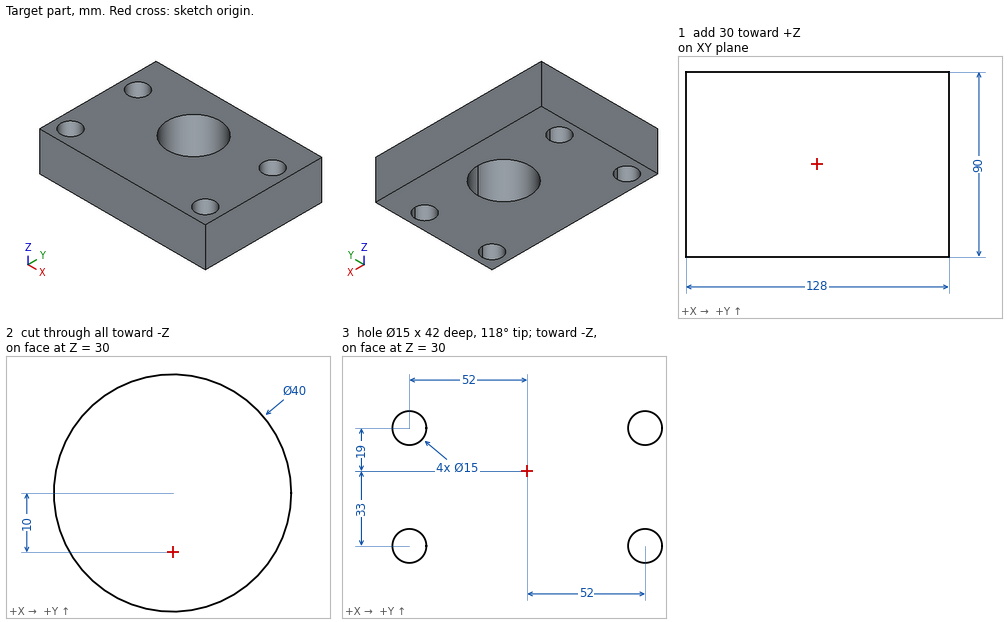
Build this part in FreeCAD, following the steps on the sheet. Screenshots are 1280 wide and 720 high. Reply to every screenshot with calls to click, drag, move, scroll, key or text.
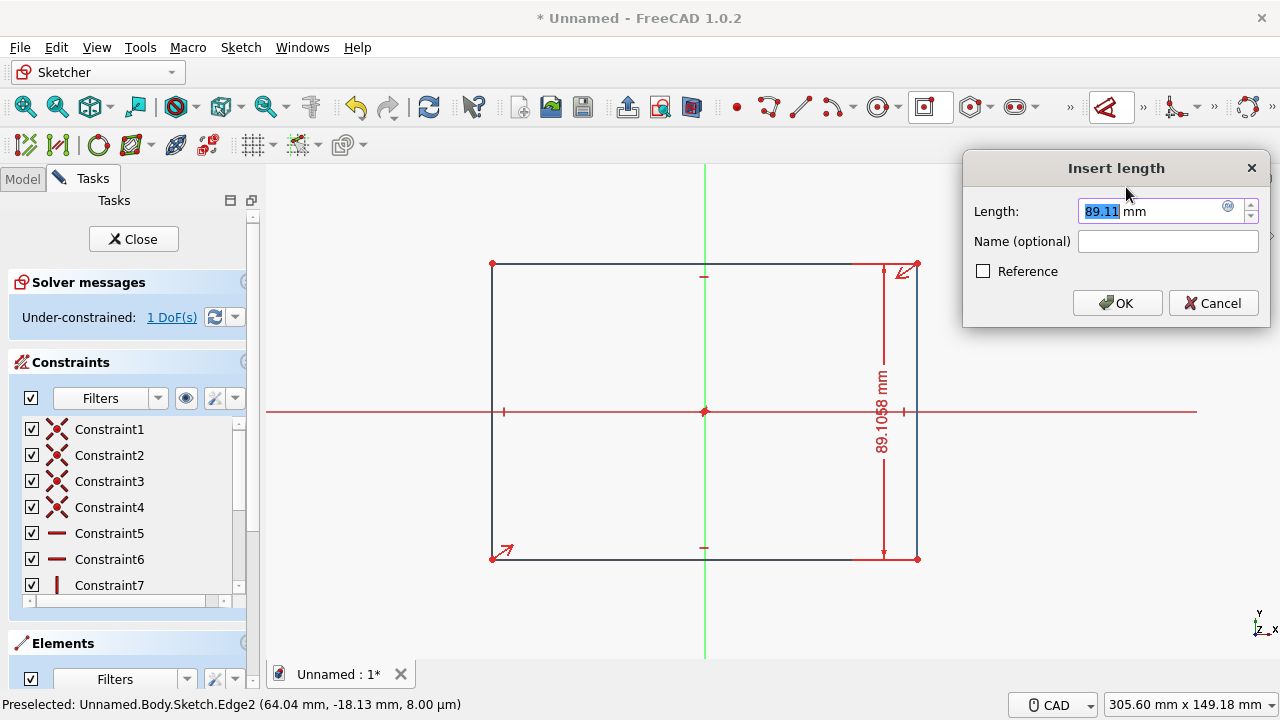
text(90)
key(Return)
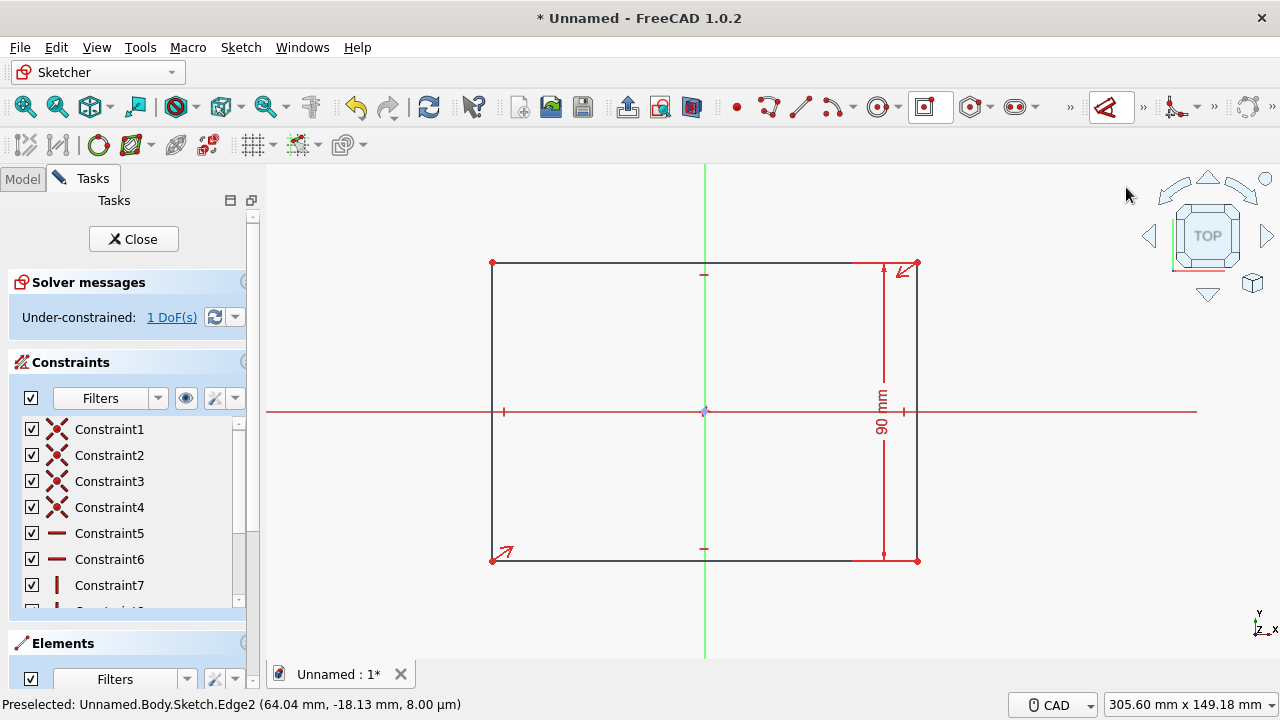
click(620, 561)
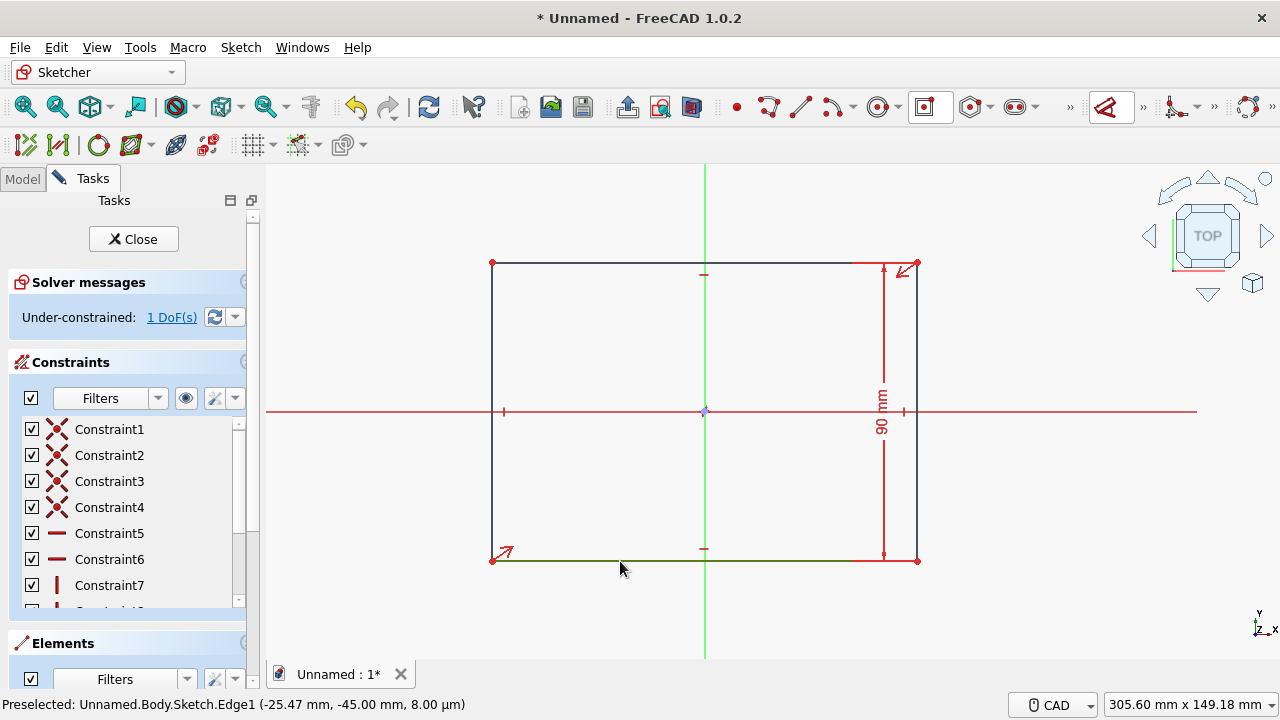
click(1128, 108)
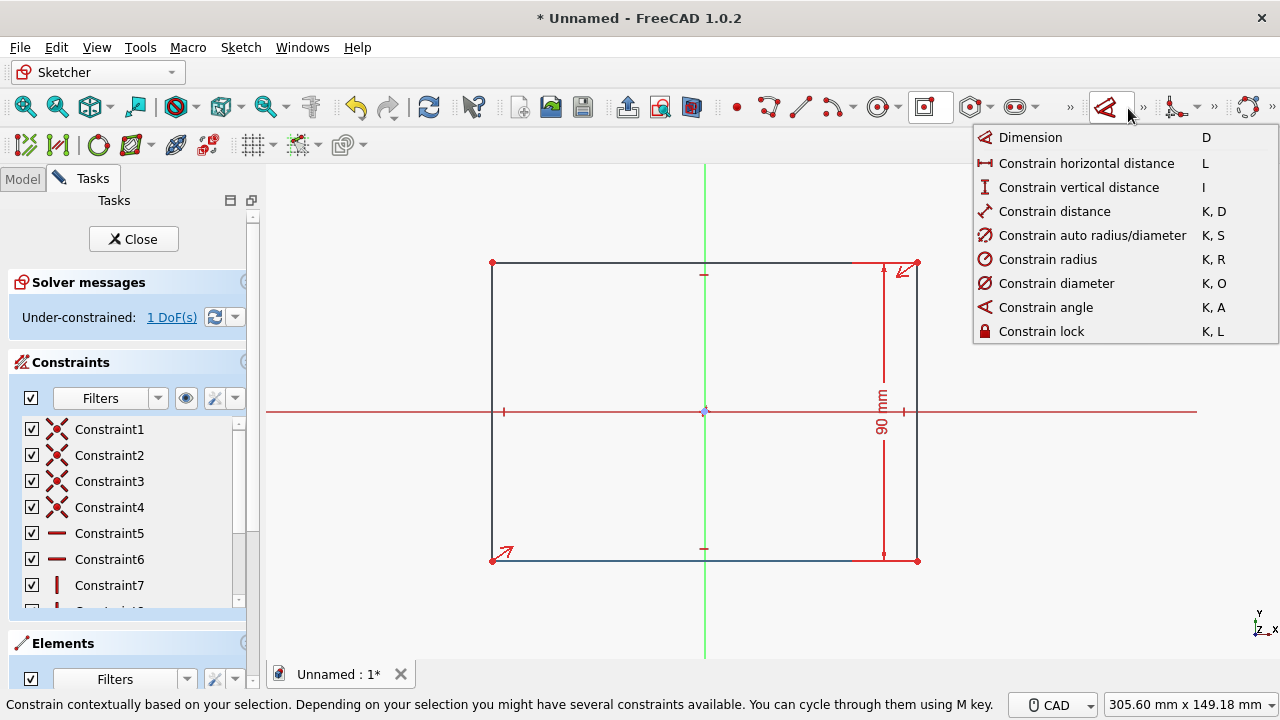
click(1126, 163)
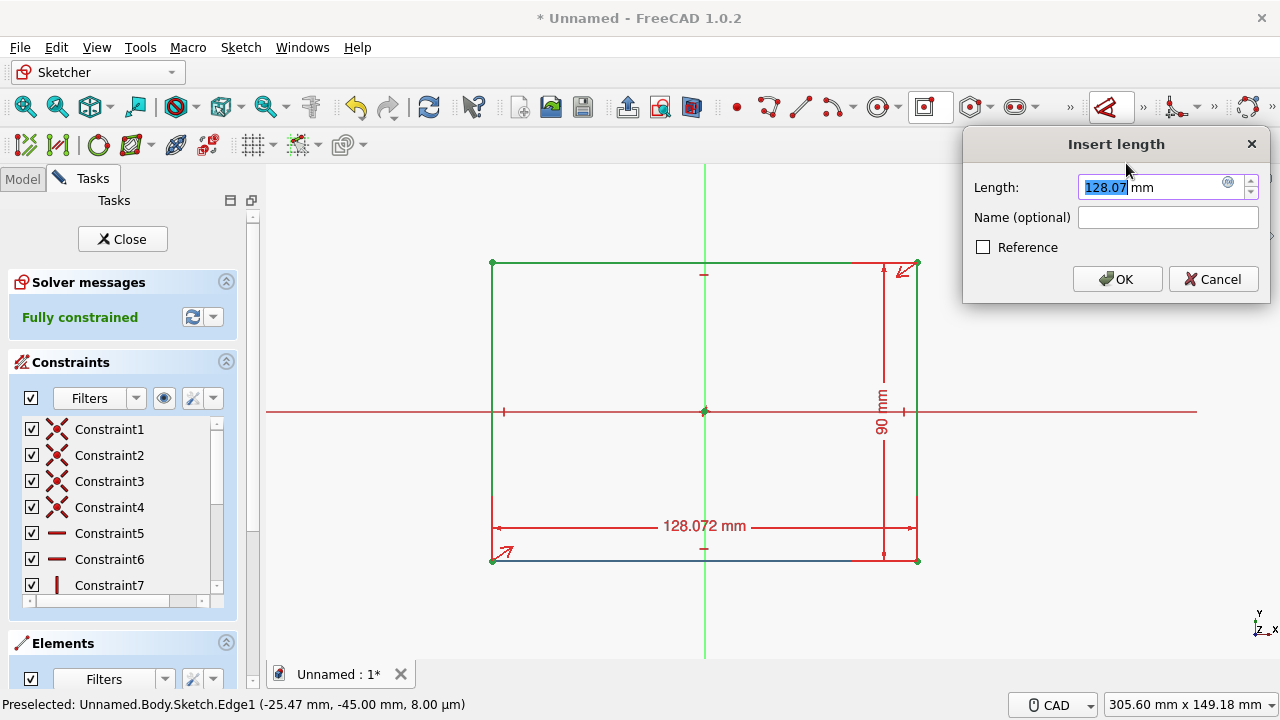
text(128)
key(Return)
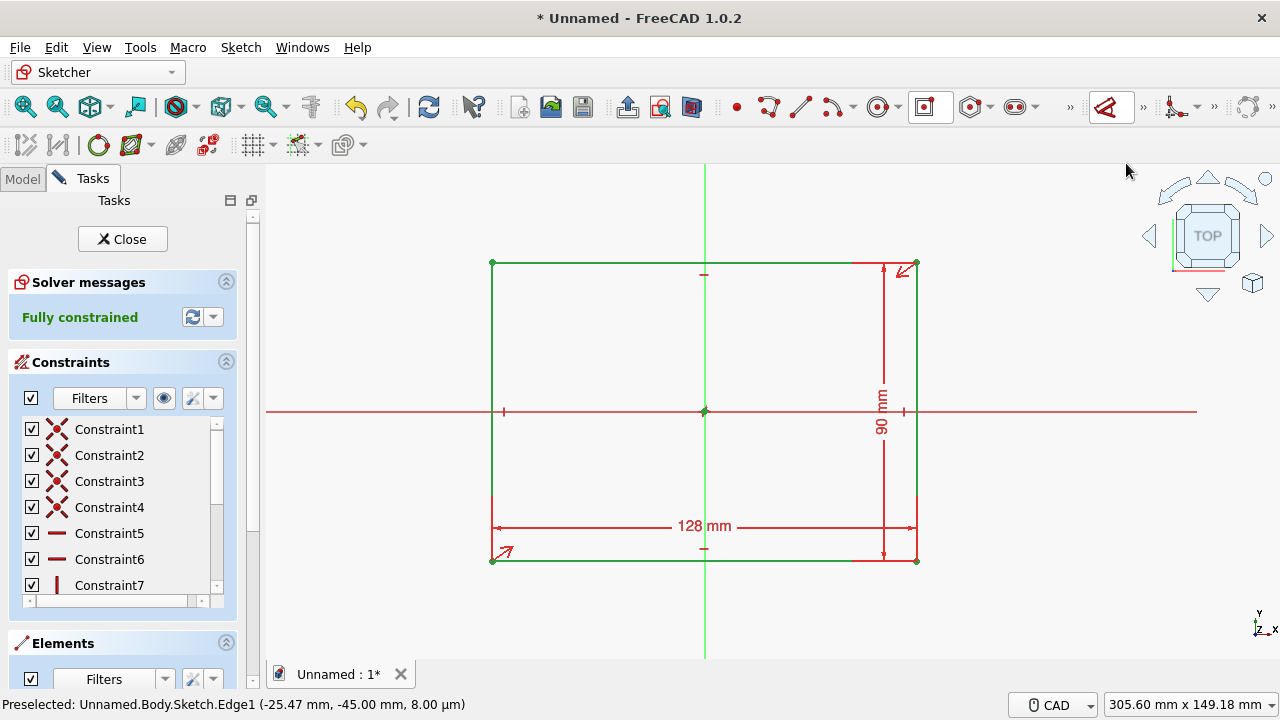
click(123, 239)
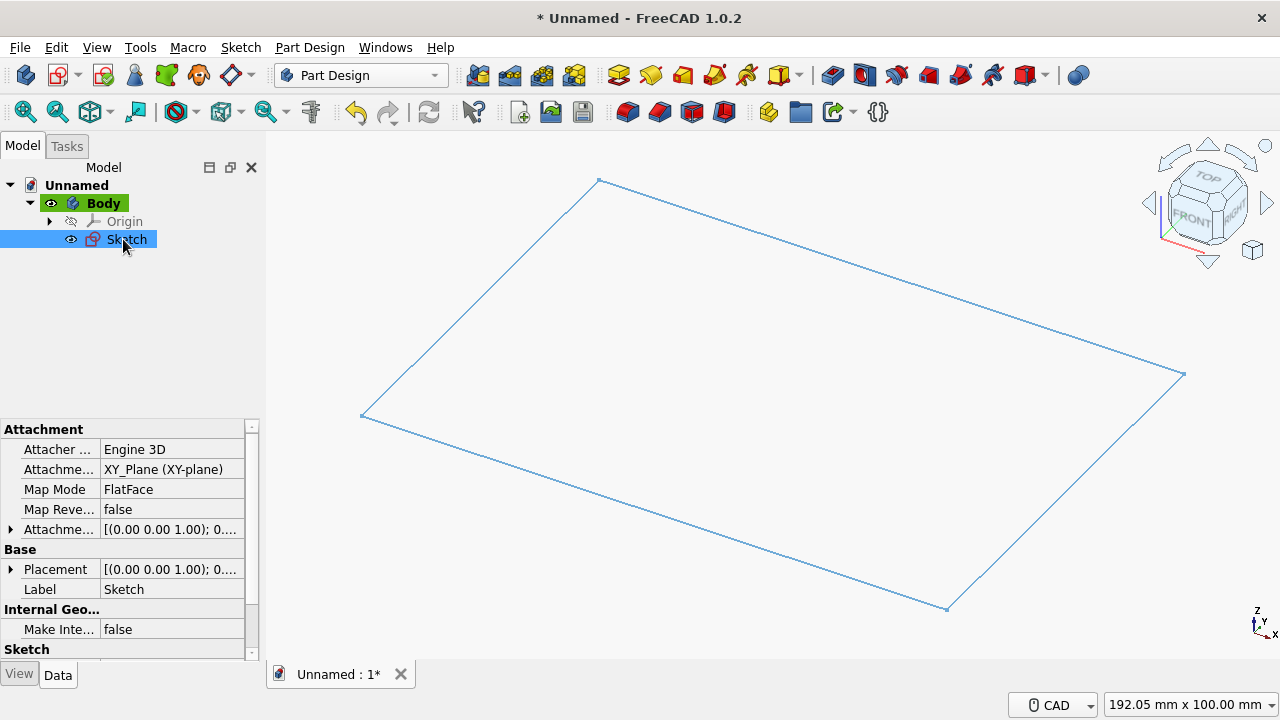
click(620, 76)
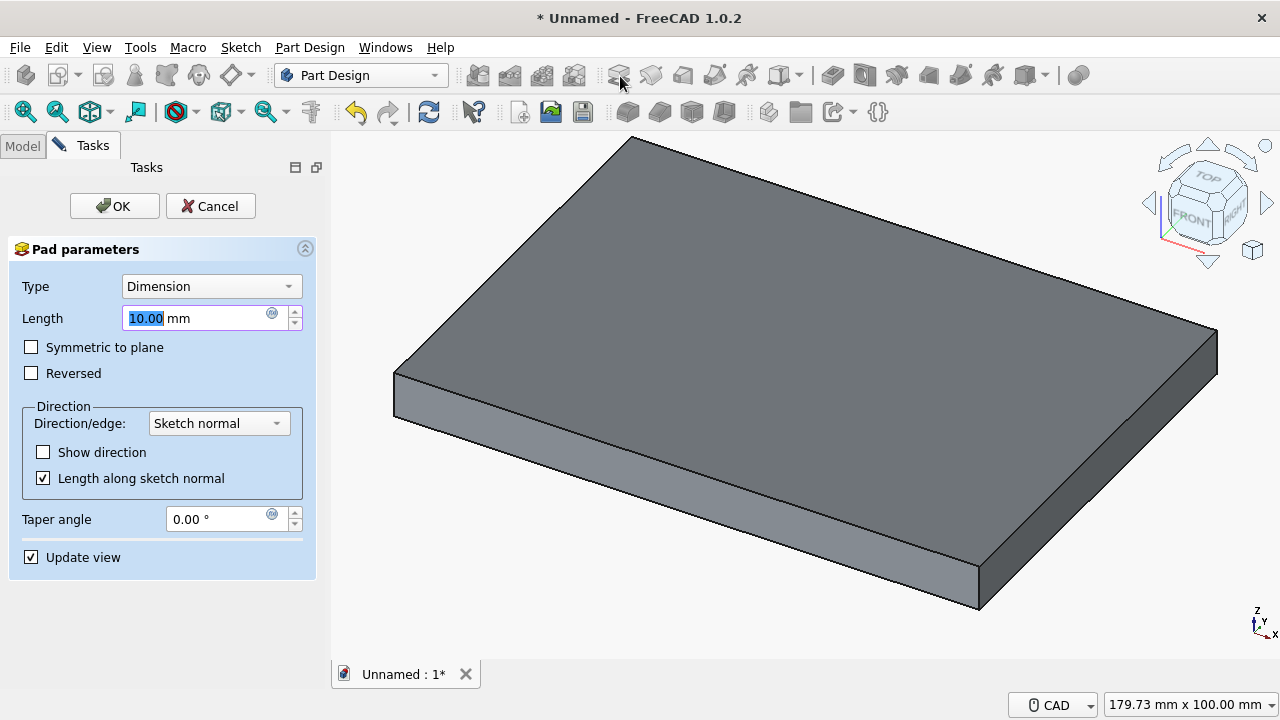
text(30)
key(Tab)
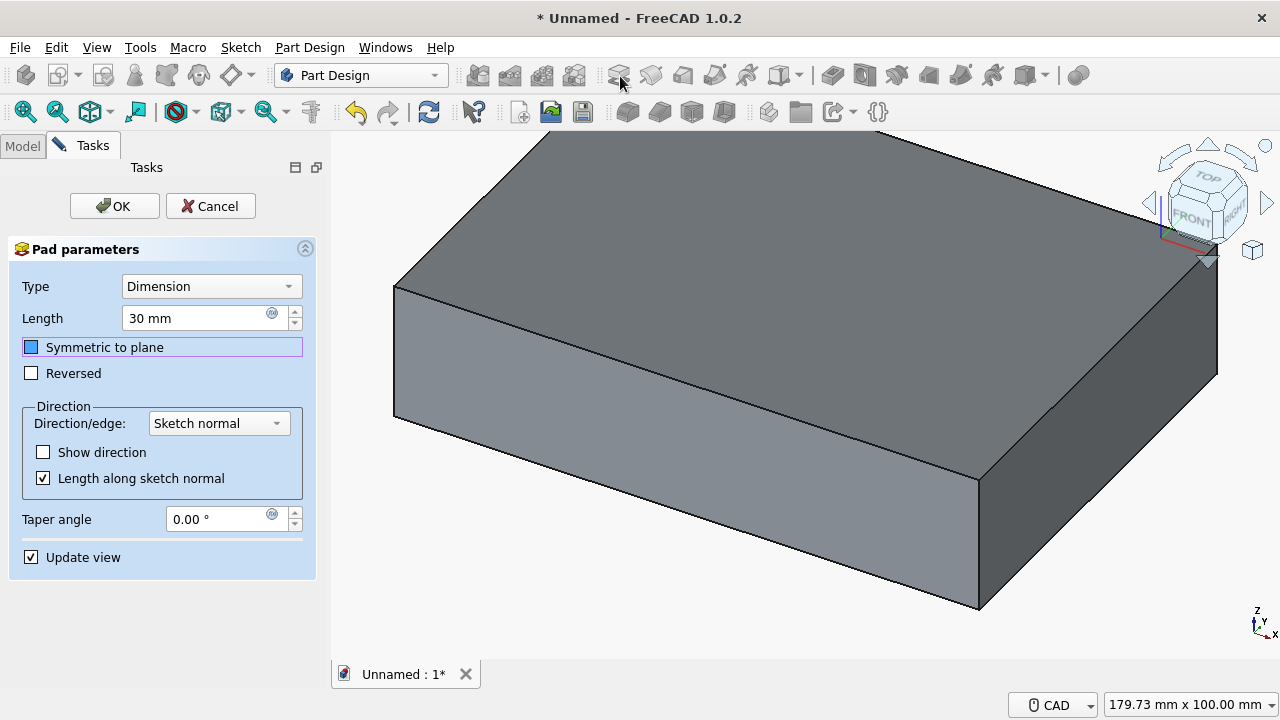
click(115, 206)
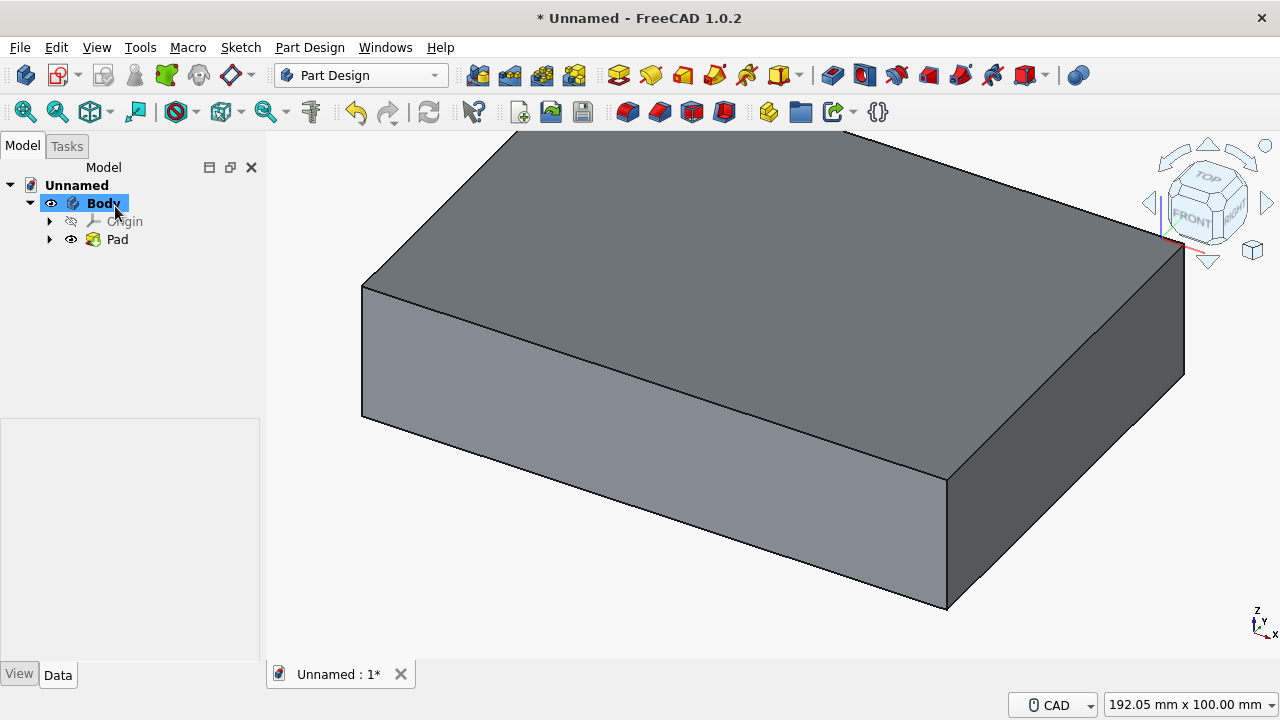
key(v)
key(f)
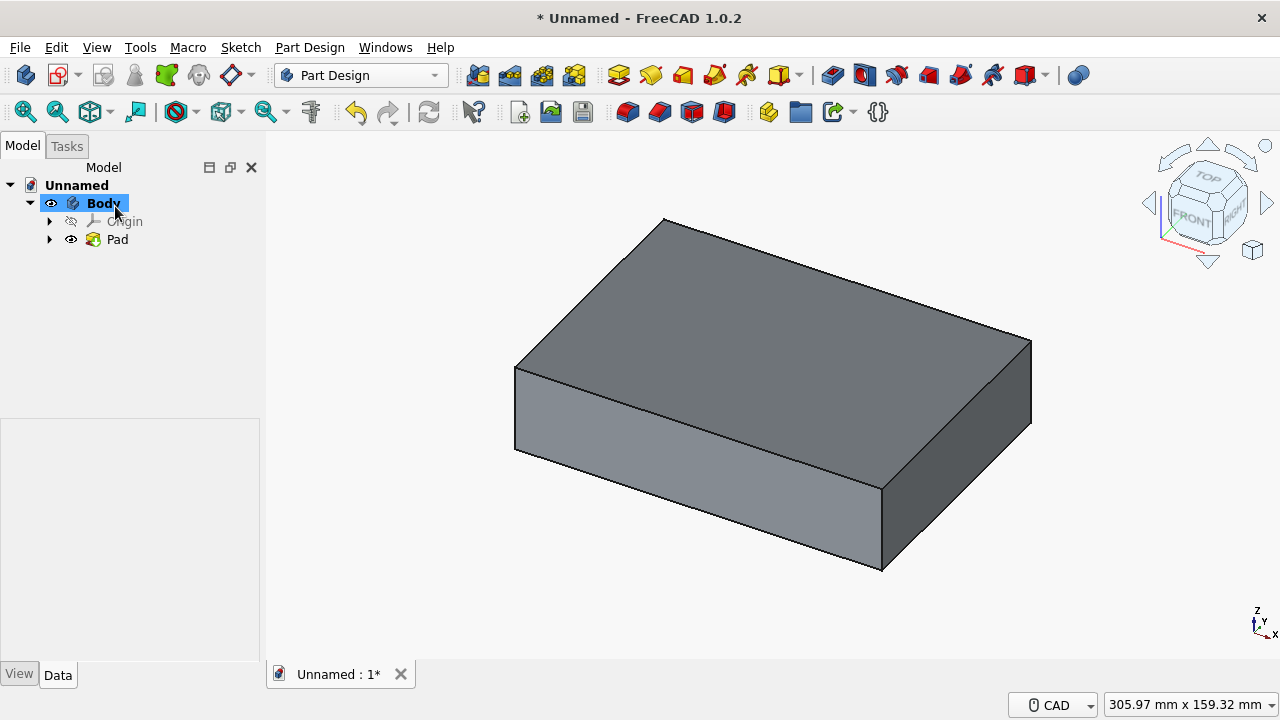
click(825, 371)